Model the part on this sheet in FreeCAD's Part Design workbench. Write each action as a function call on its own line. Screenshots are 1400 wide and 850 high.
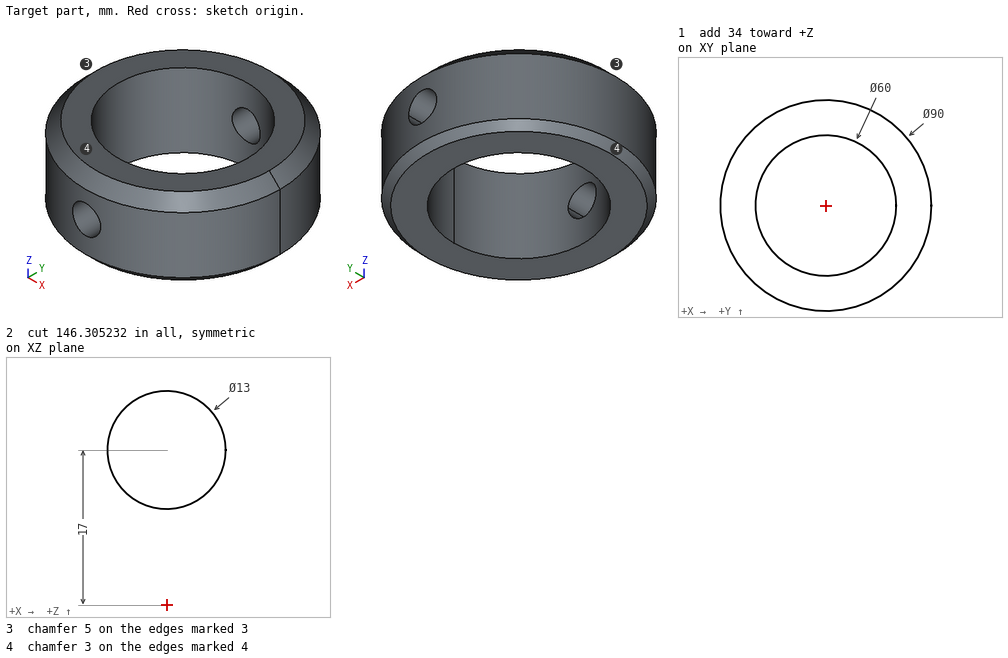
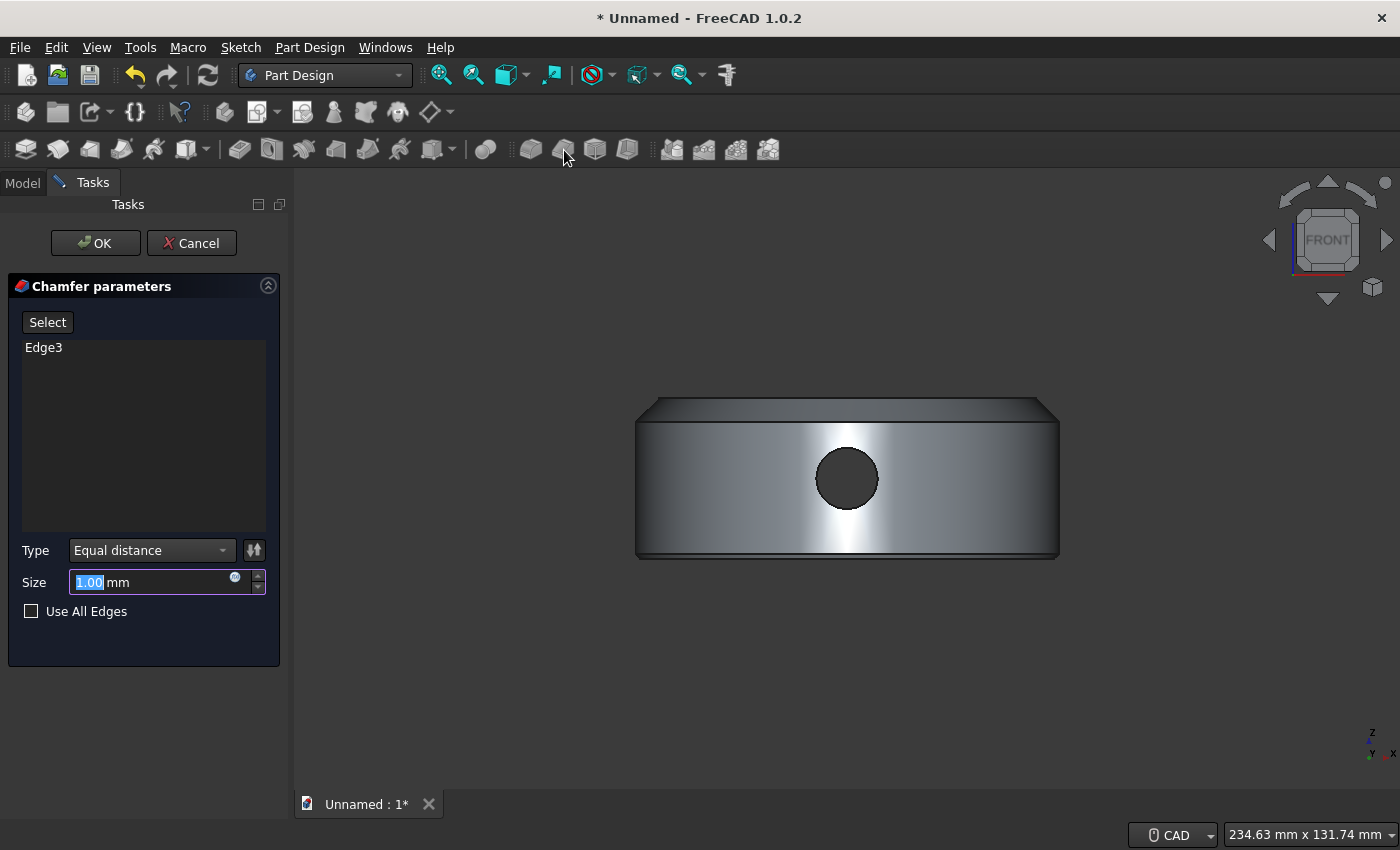
text(3)
key(Tab)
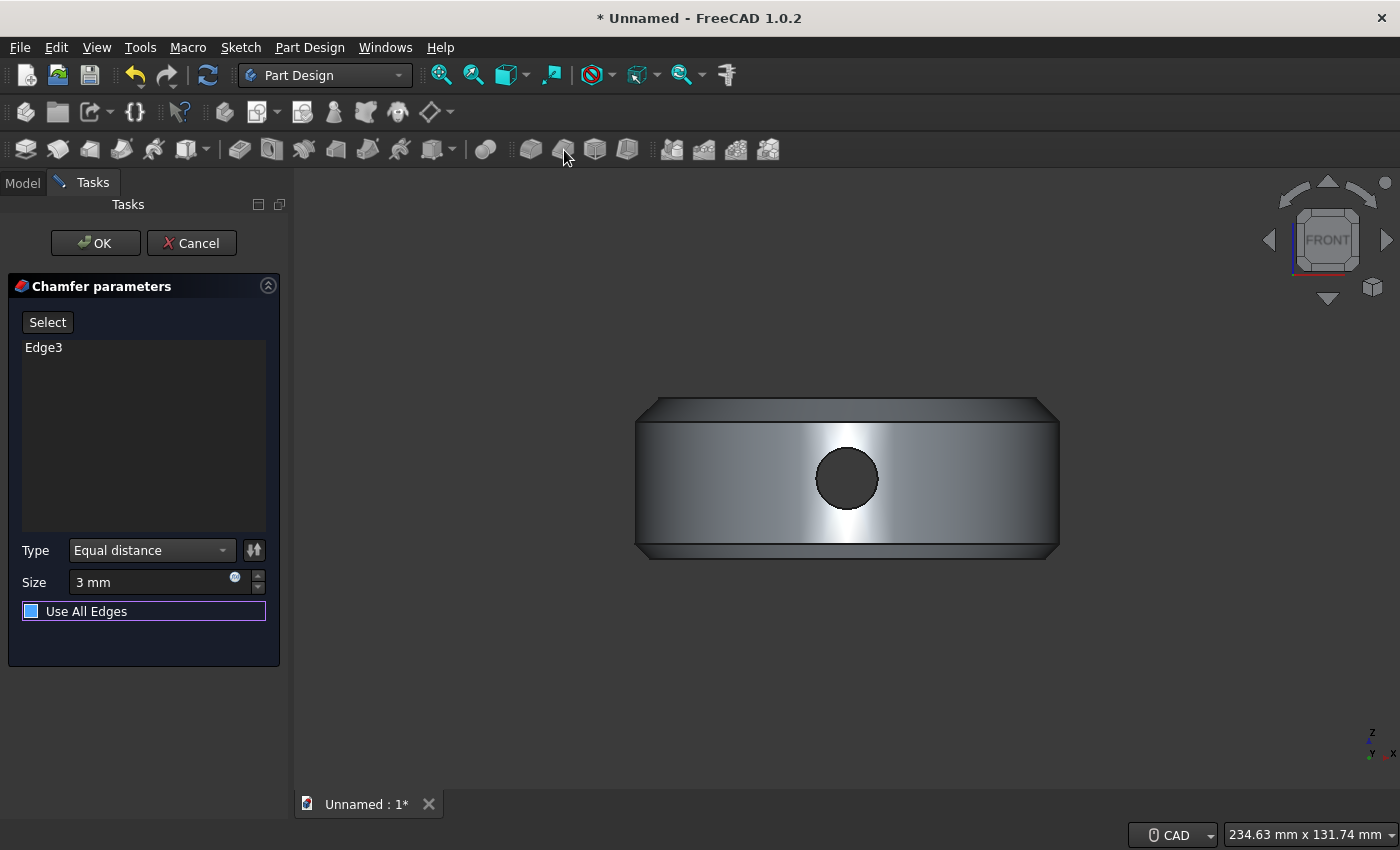
click(96, 243)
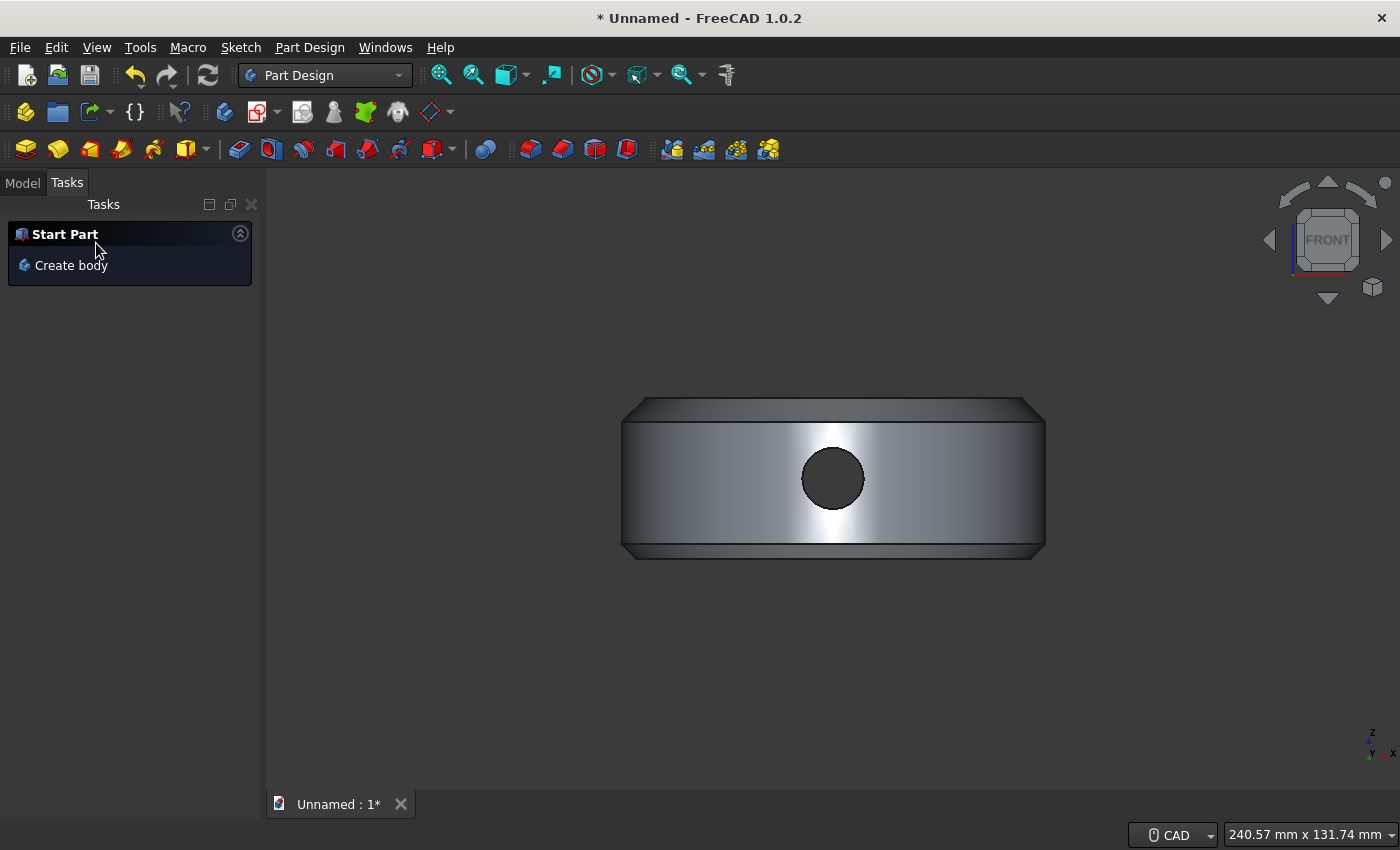
key(0)